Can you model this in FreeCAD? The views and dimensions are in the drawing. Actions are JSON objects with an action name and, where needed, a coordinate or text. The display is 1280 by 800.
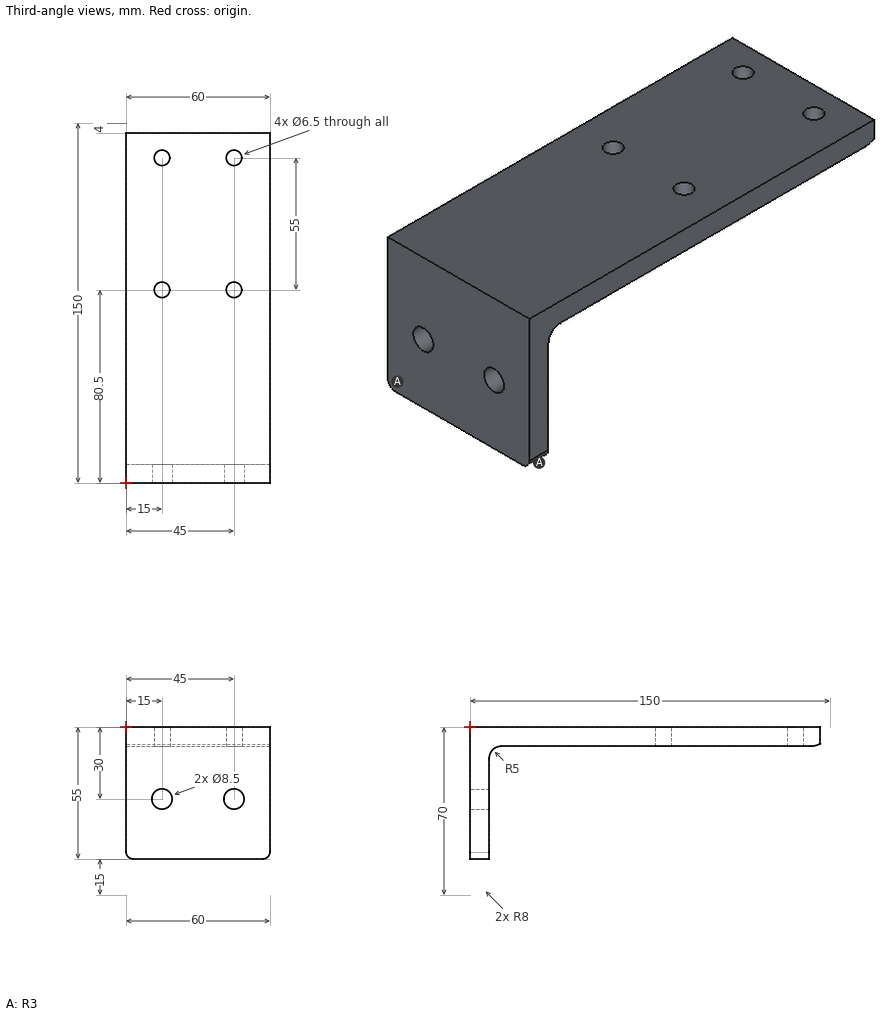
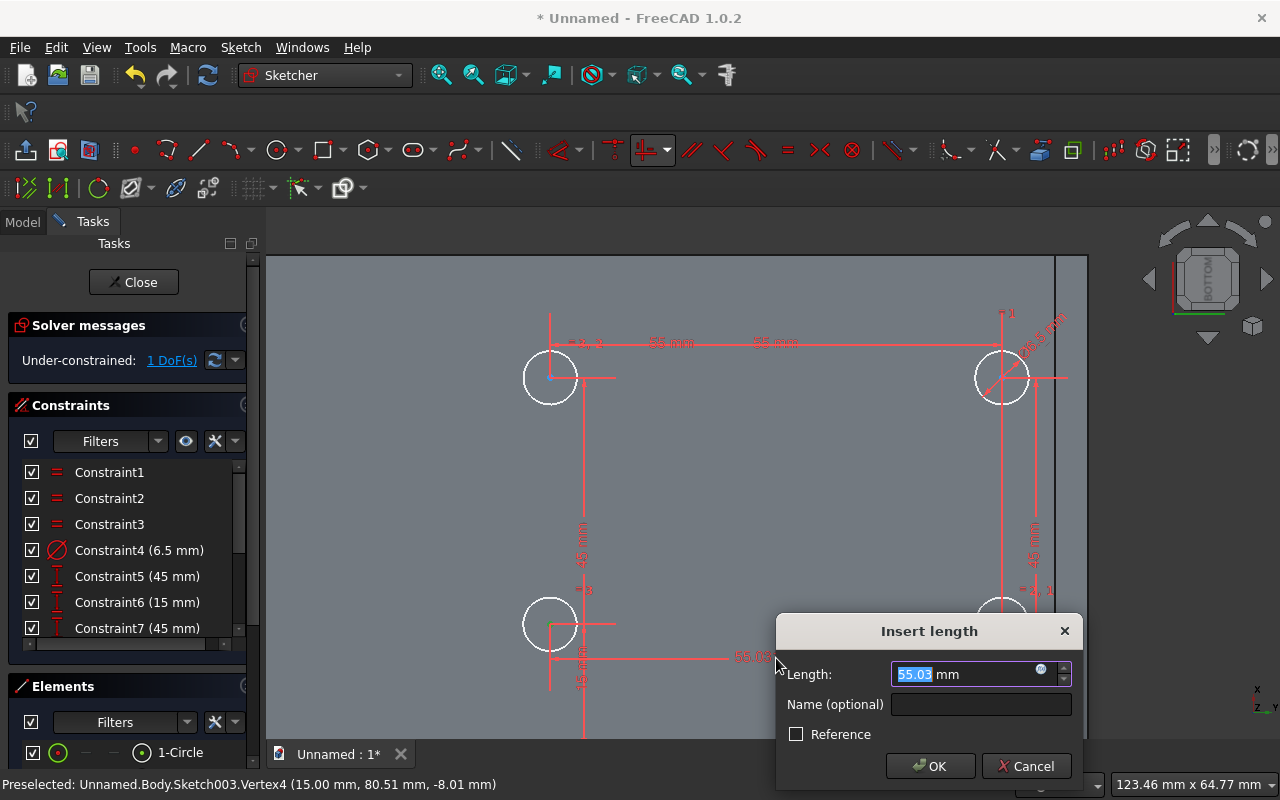
{"action": "type", "text": "55"}
{"action": "key", "text": "Return"}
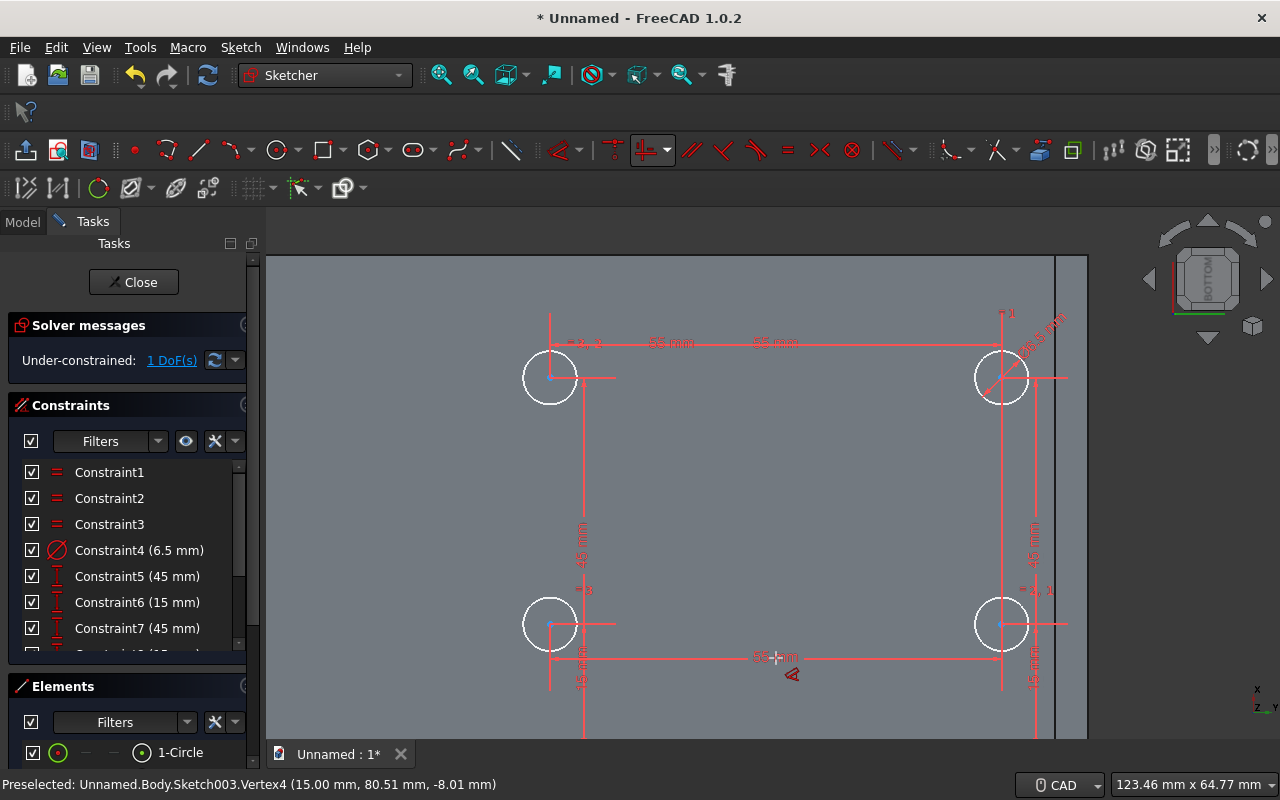
{"action": "left_click", "coordinate": [550, 378]}
{"action": "left_click", "coordinate": [422, 344]}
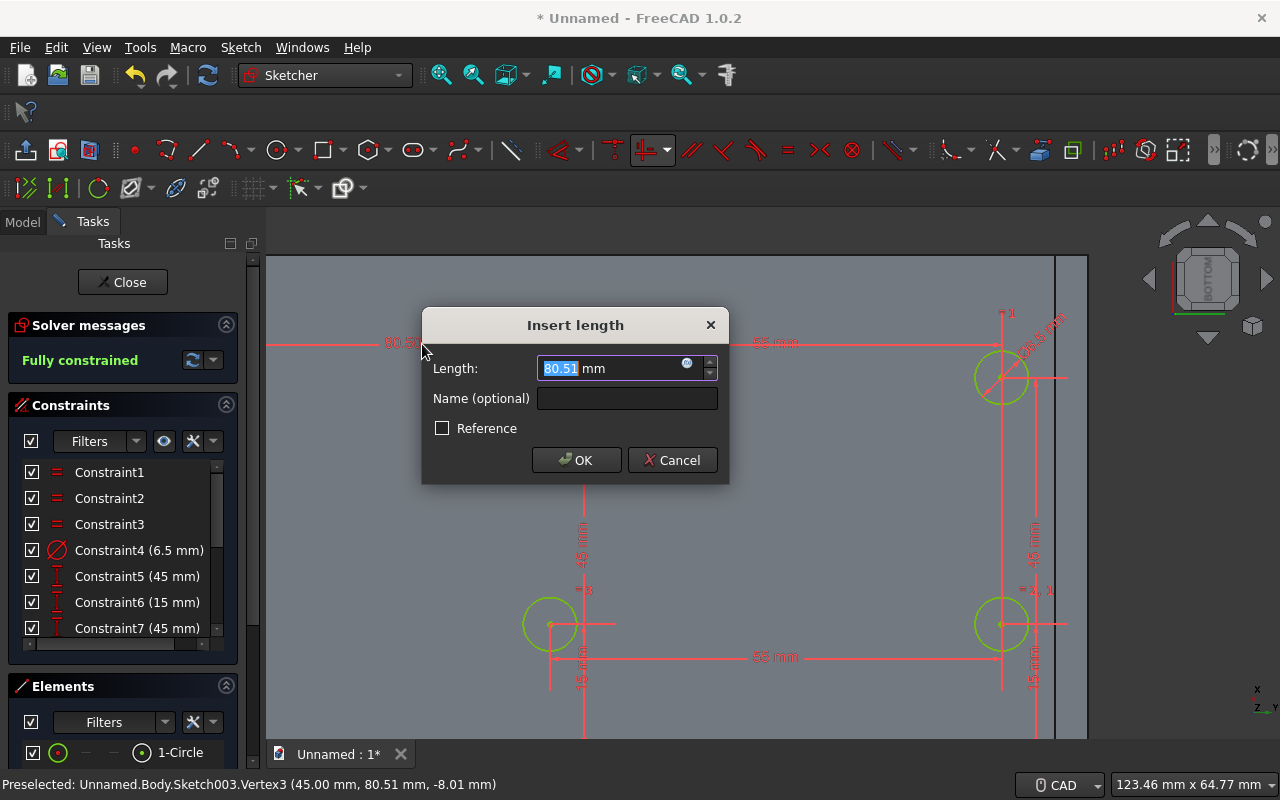
{"action": "type", "text": "80.5"}
{"action": "key", "text": "Return"}
{"action": "key", "text": "Escape"}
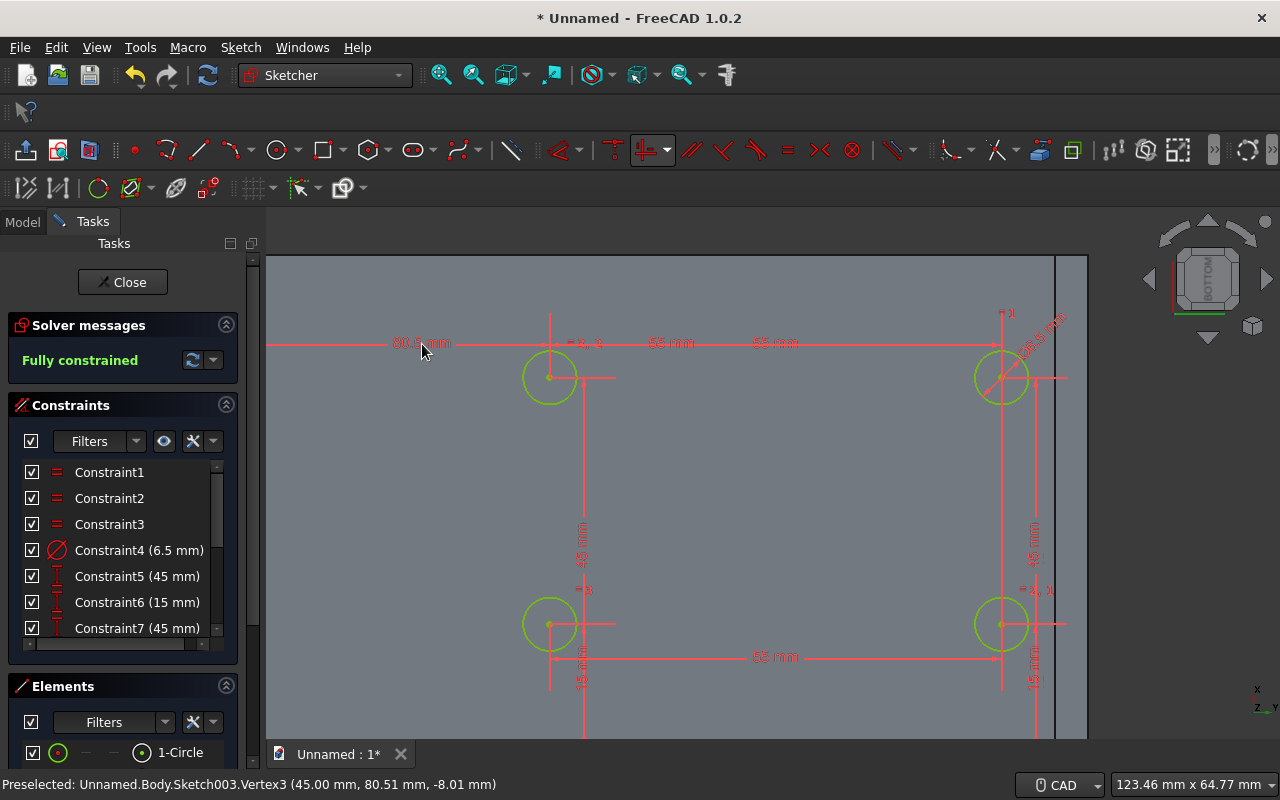
{"action": "left_click", "coordinate": [123, 282]}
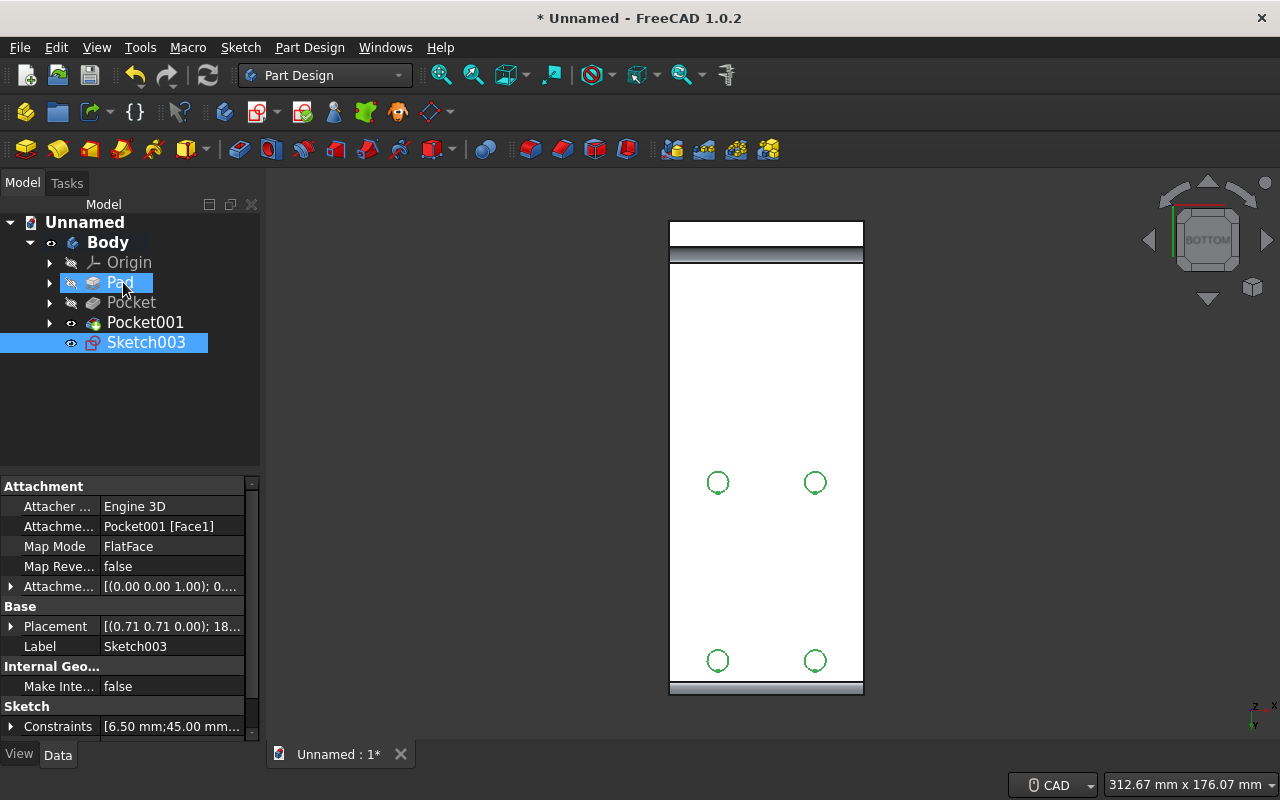
{"action": "left_click", "coordinate": [272, 150]}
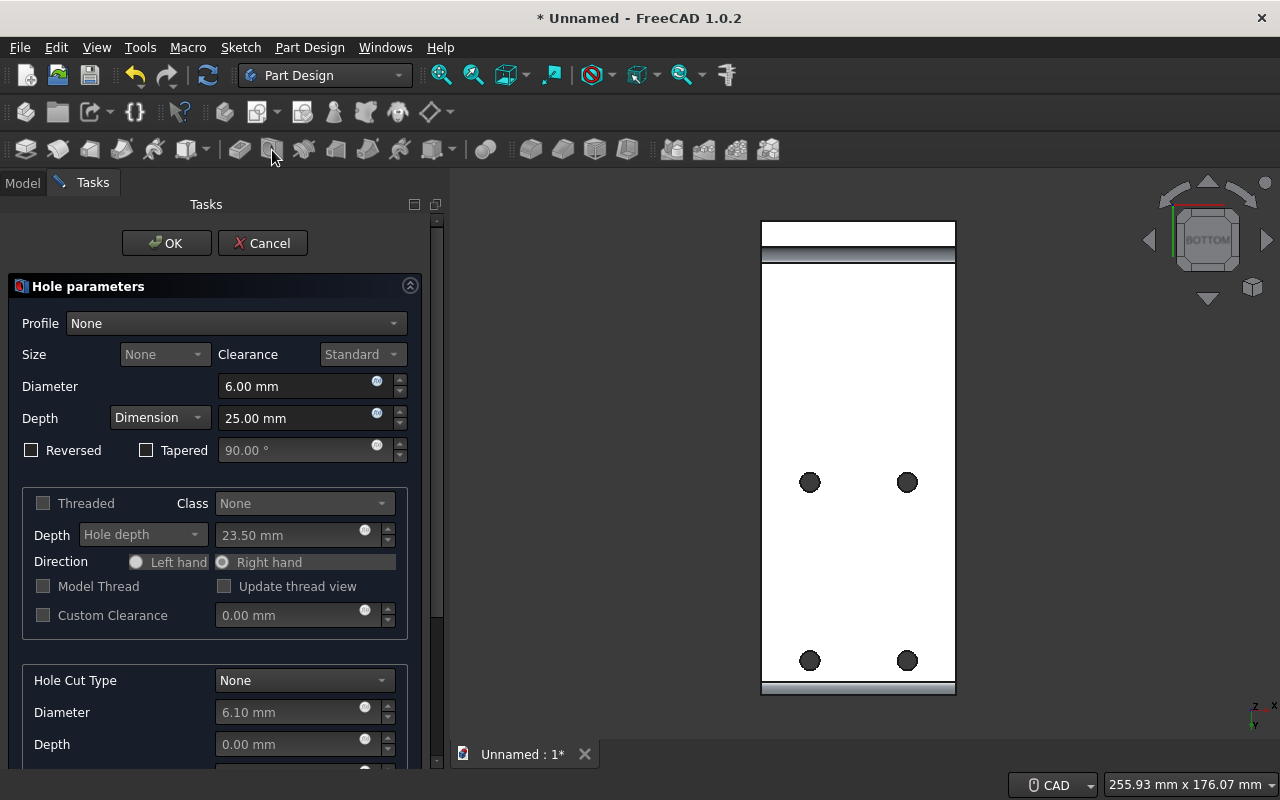
{"action": "triple_click", "coordinate": [305, 386]}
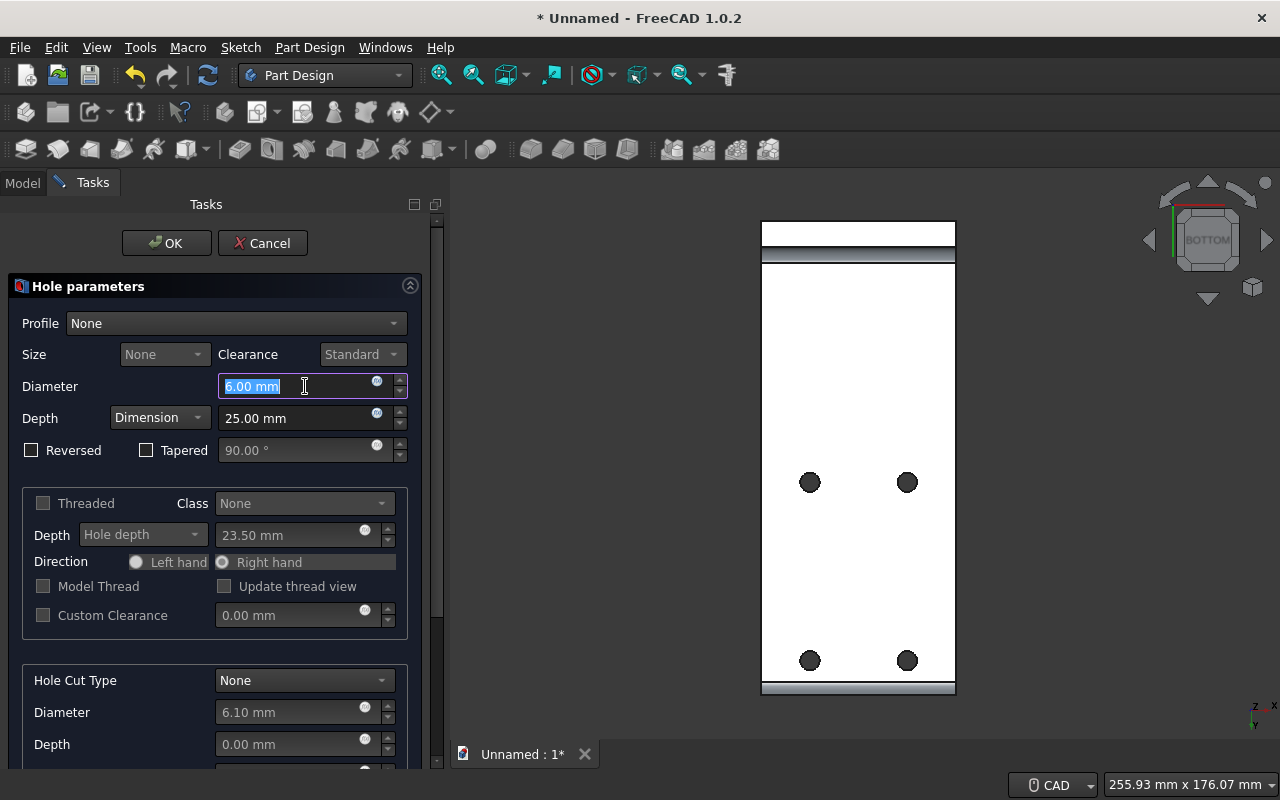
{"action": "type", "text": "6.5"}
{"action": "key", "text": "Tab"}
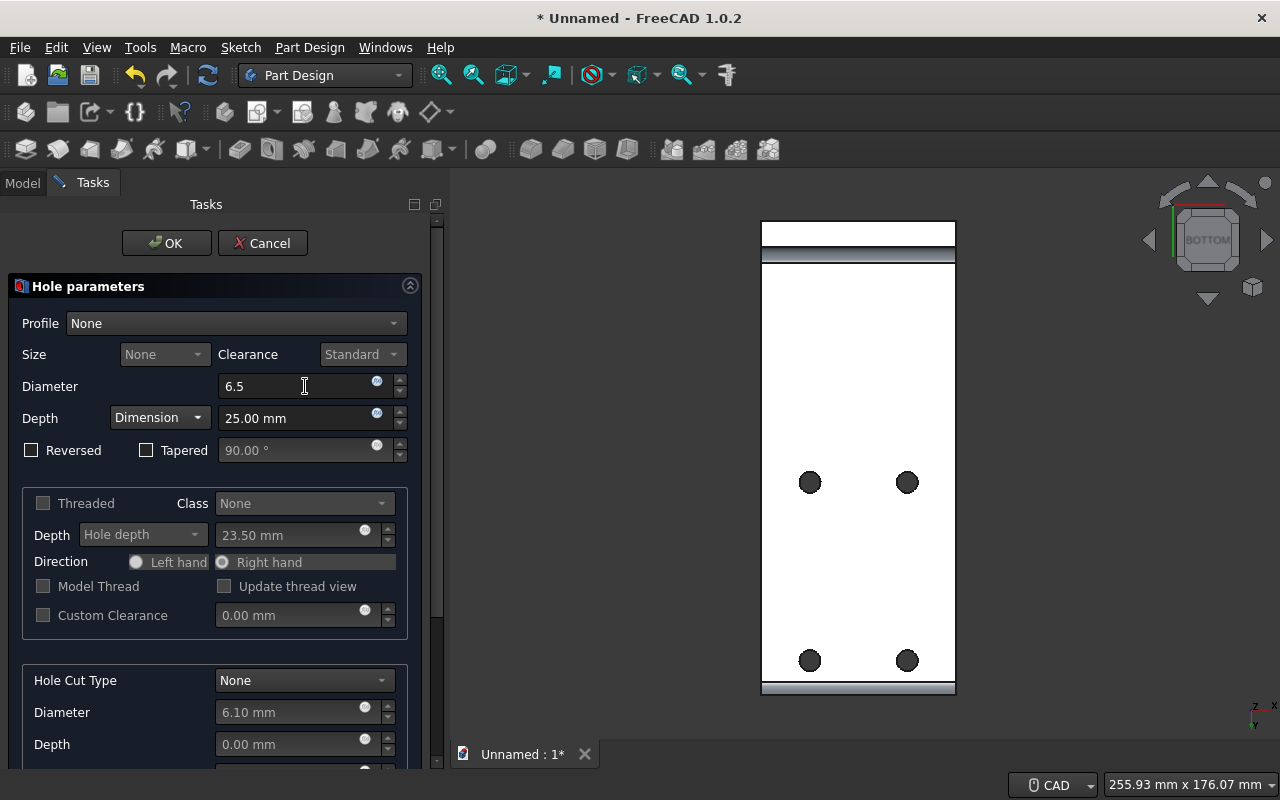
{"action": "left_click", "coordinate": [161, 418]}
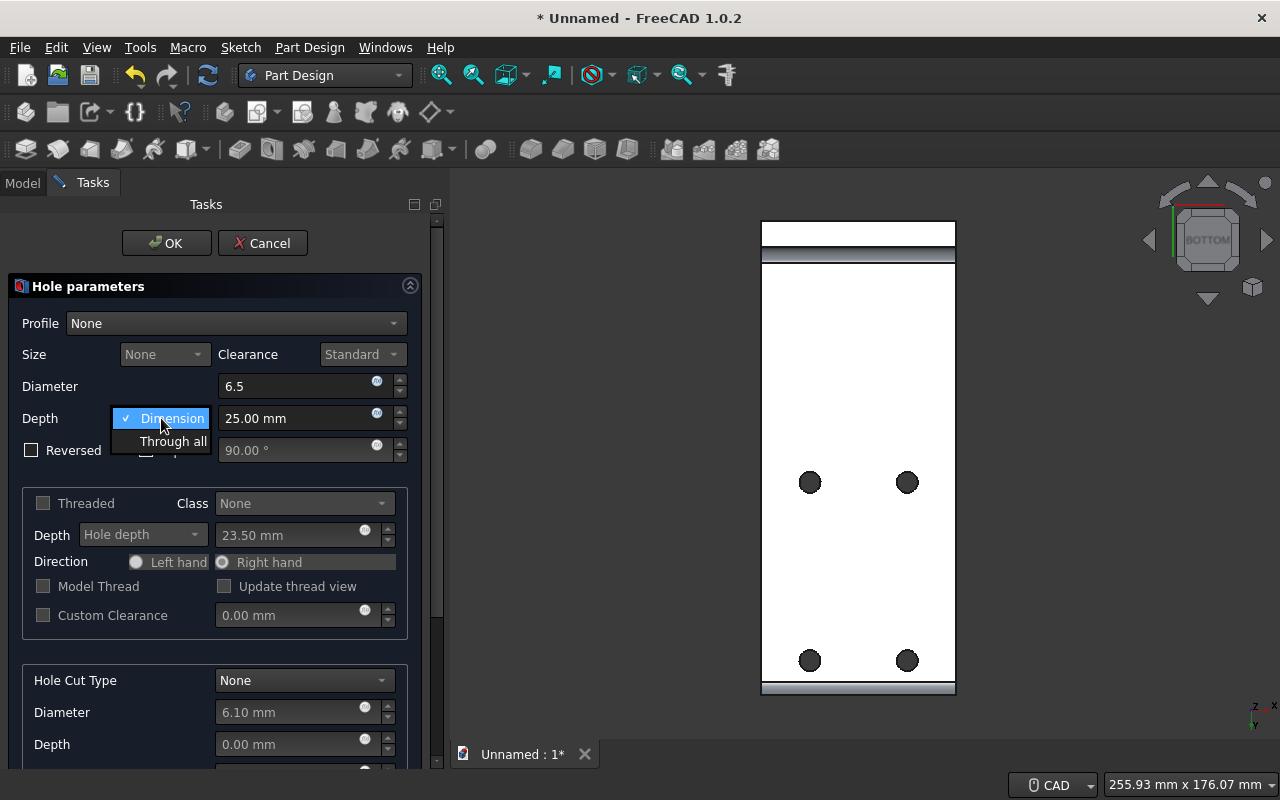
{"action": "left_click", "coordinate": [160, 442]}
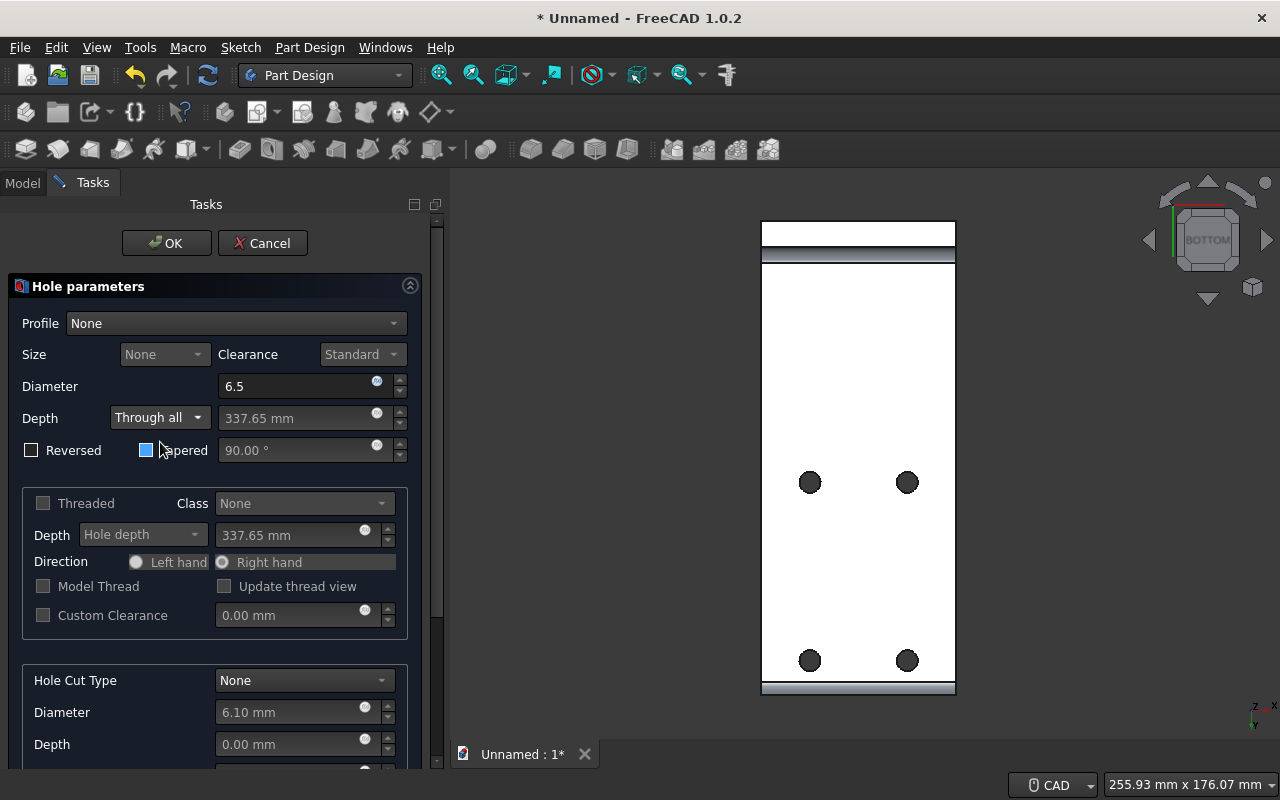
{"action": "left_click", "coordinate": [167, 243]}